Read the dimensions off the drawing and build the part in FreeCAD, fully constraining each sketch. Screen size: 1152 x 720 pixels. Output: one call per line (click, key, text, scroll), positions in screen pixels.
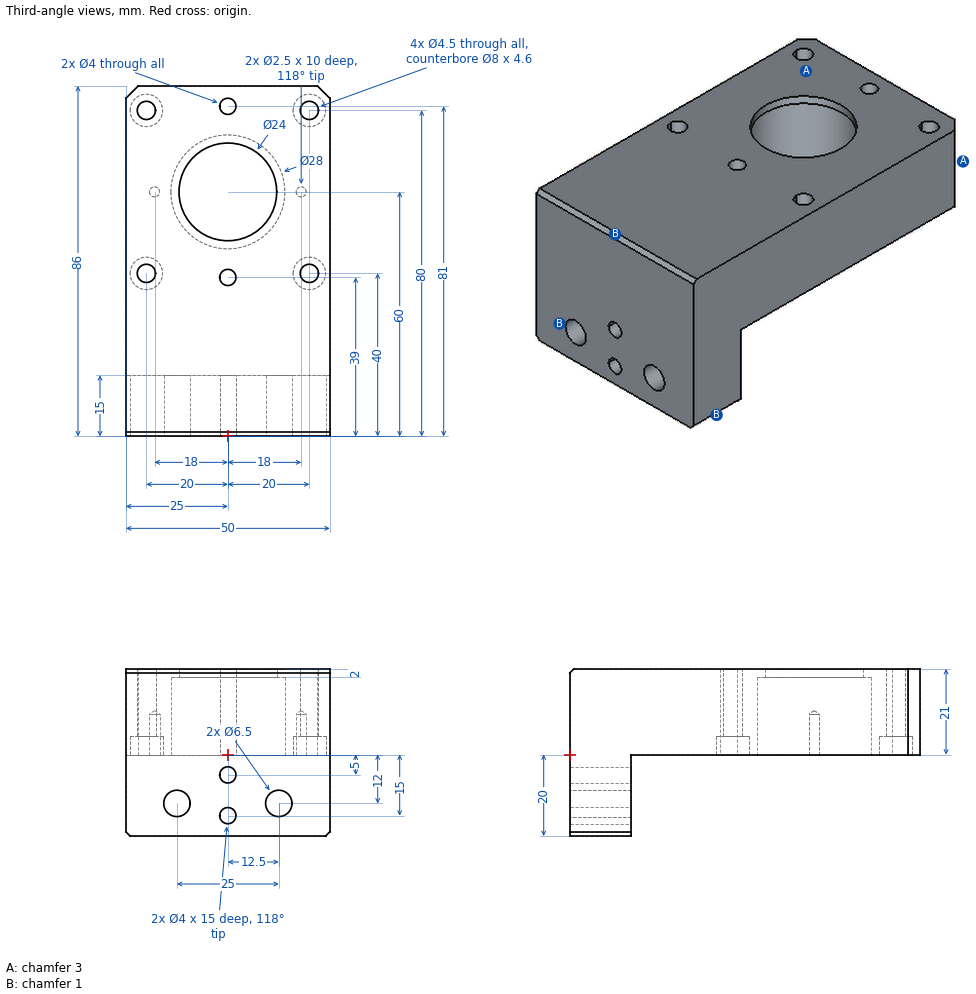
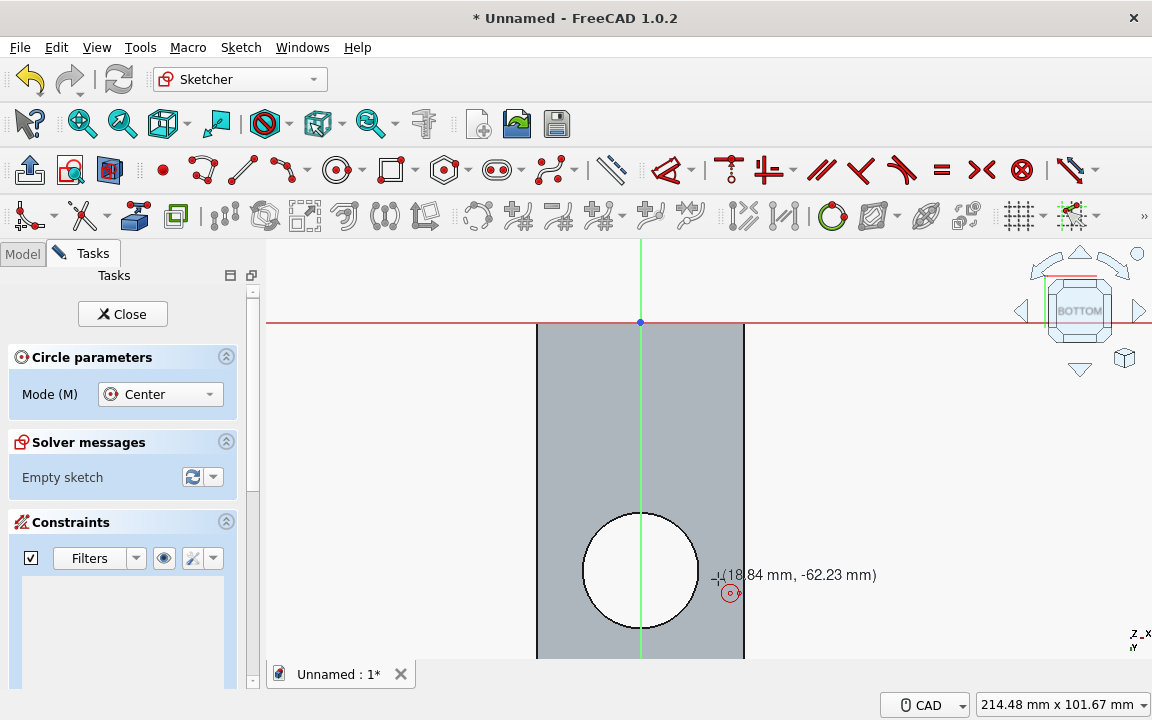
click(715, 571)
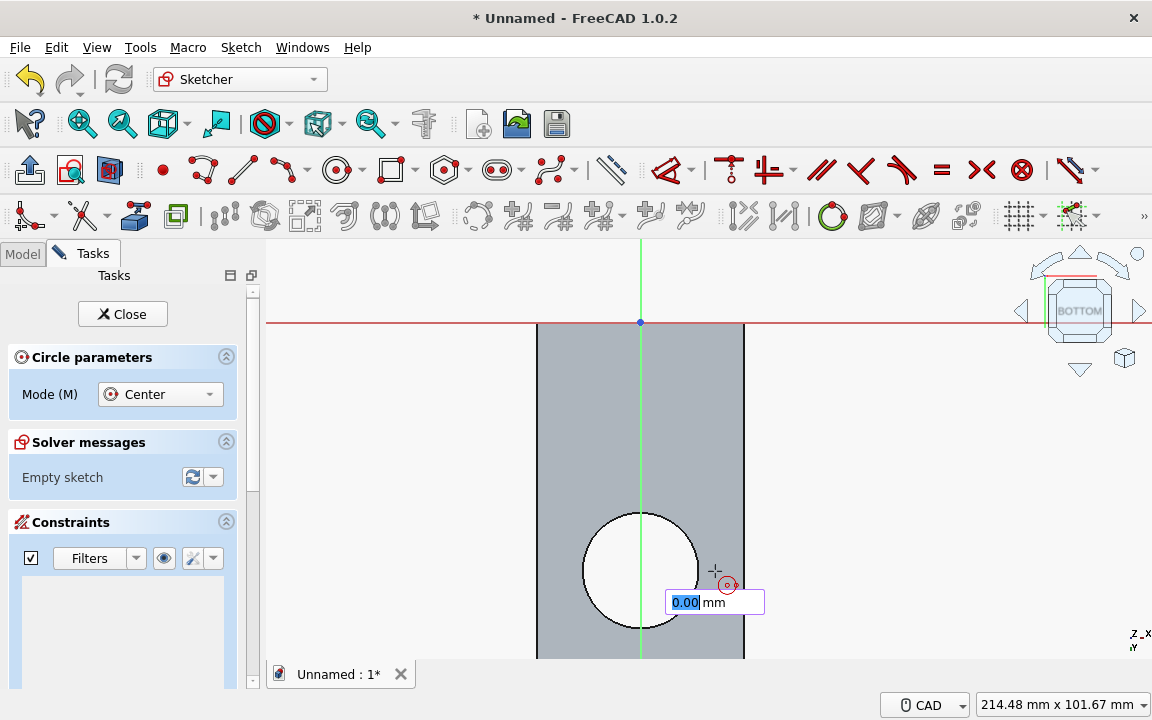
scroll(719, 567, up, 6)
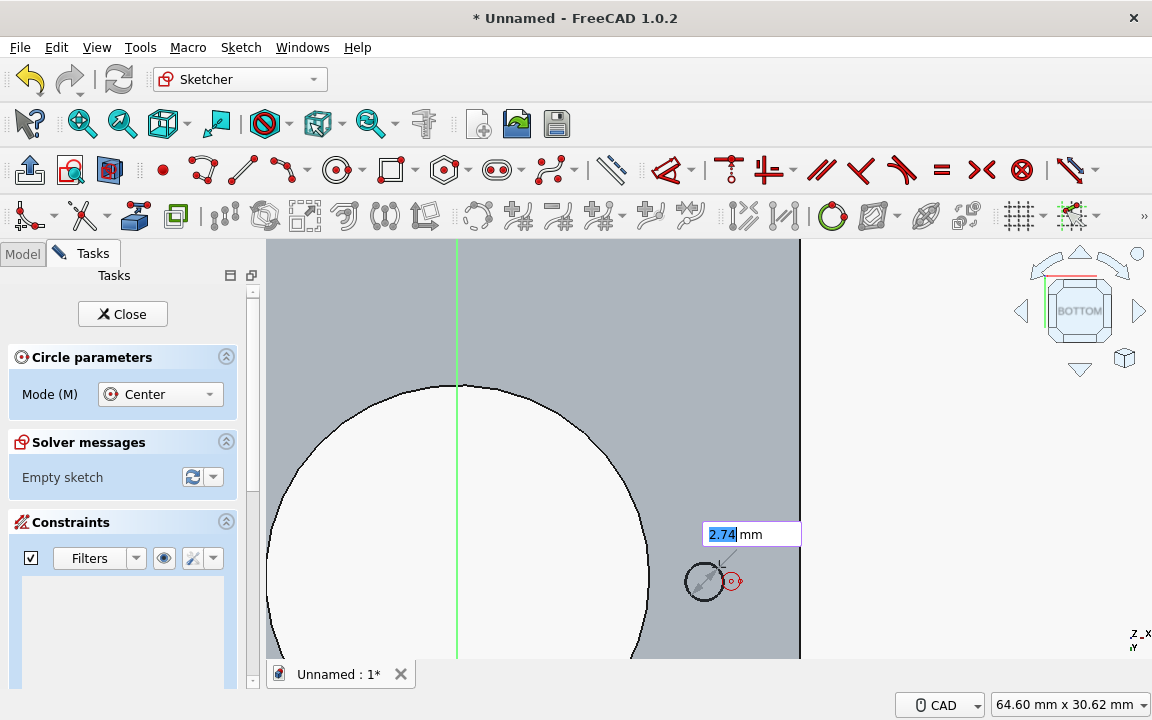
click(716, 565)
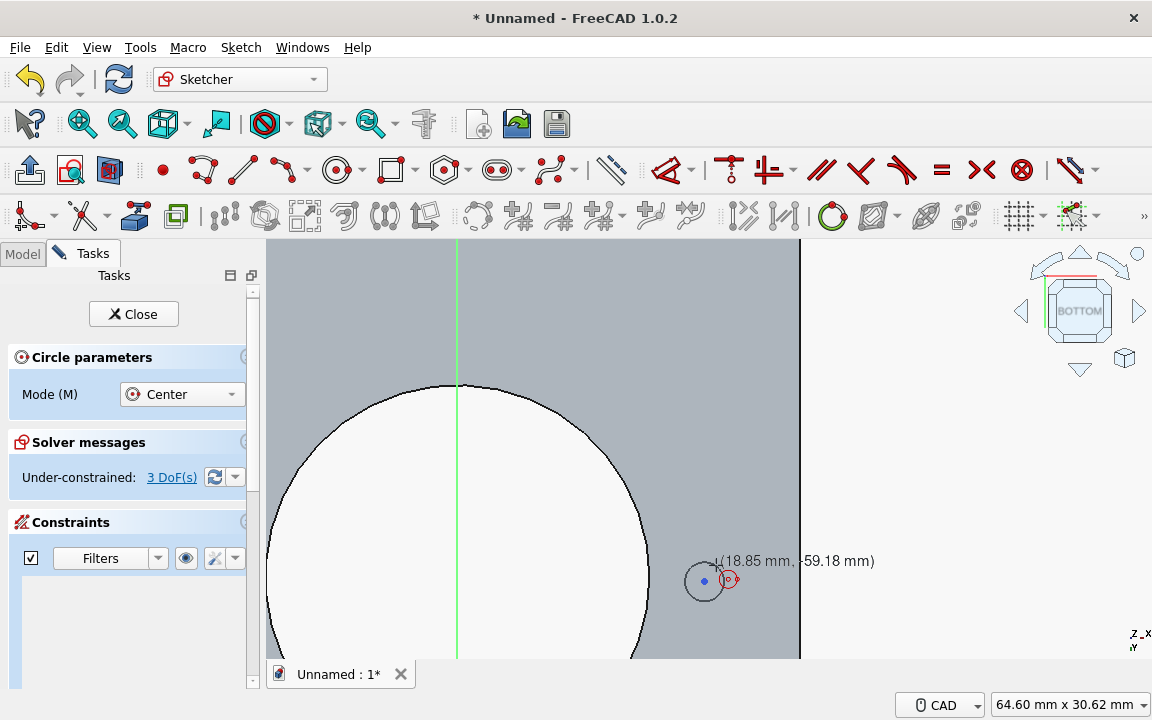
scroll(719, 567, down, 6)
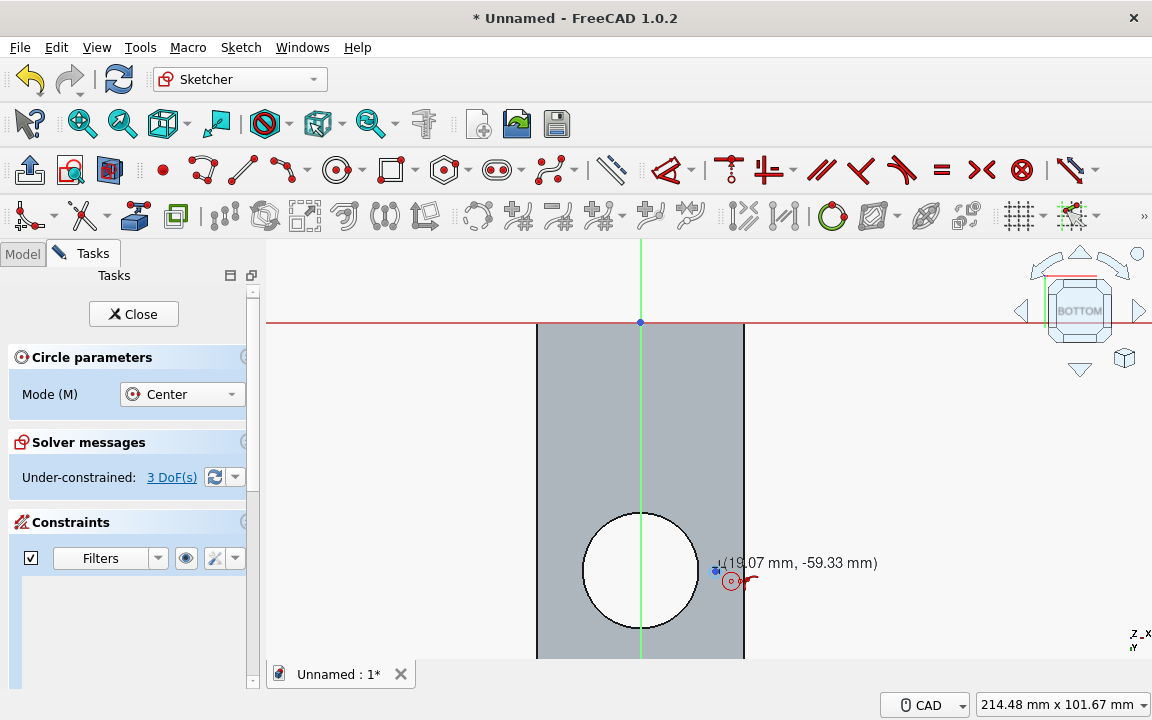
scroll(566, 571, up, 8)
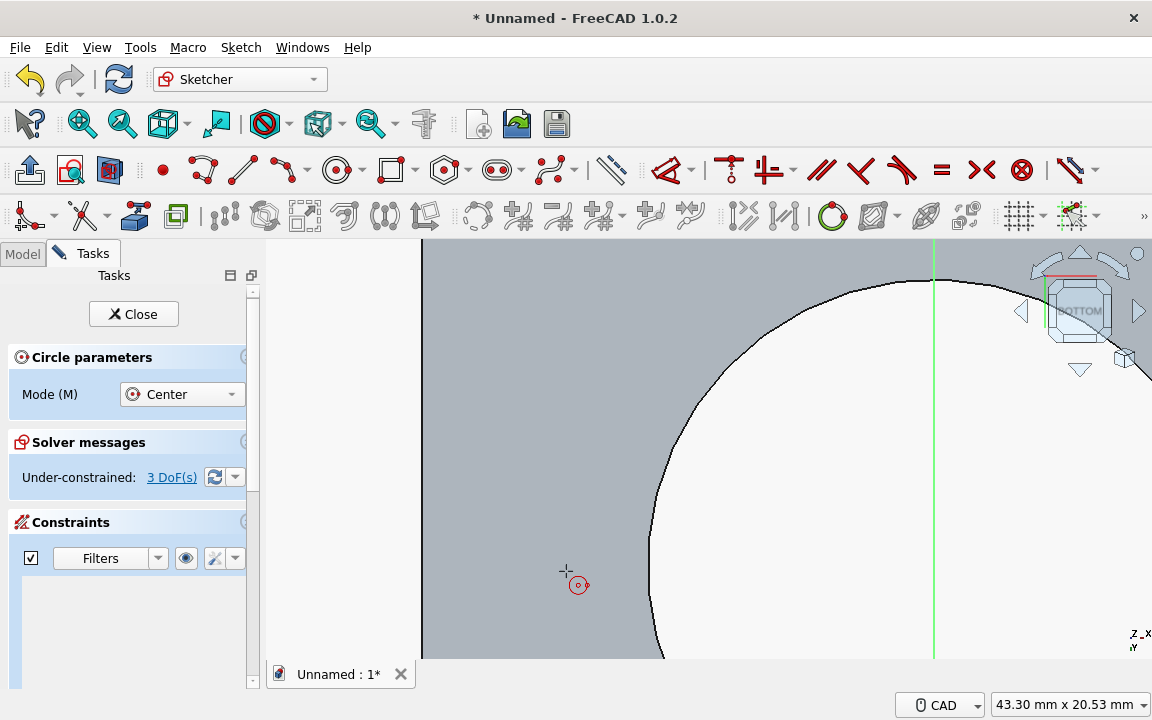
scroll(566, 571, down, 8)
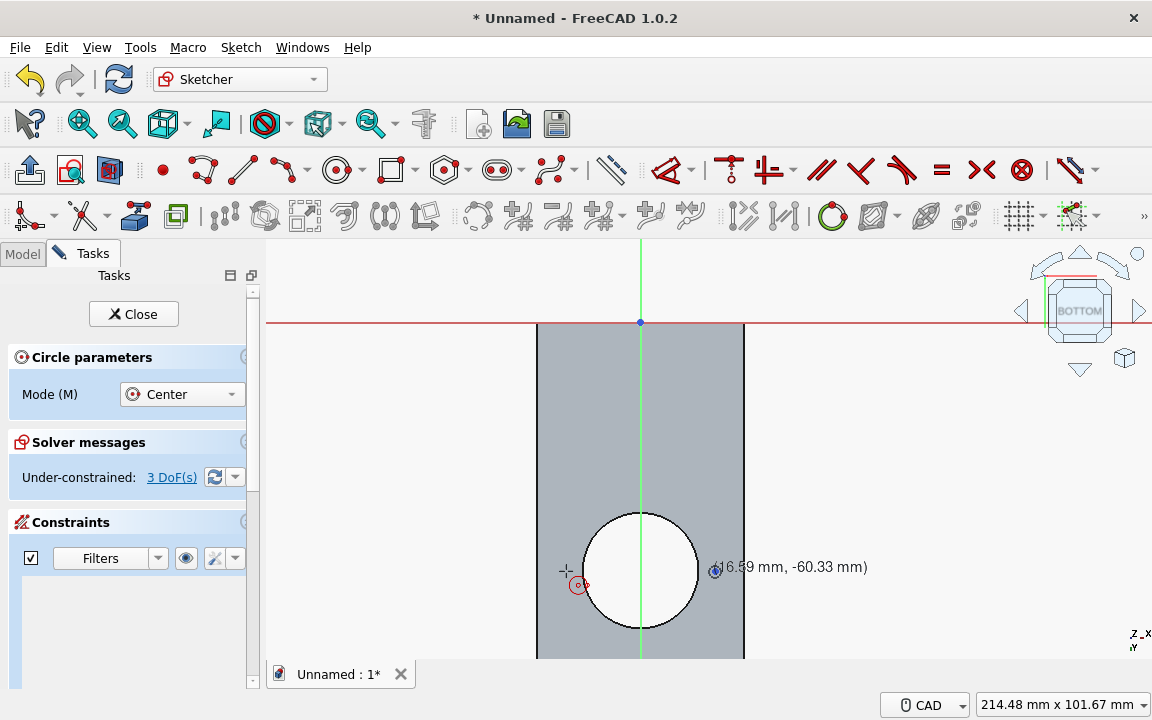
click(566, 571)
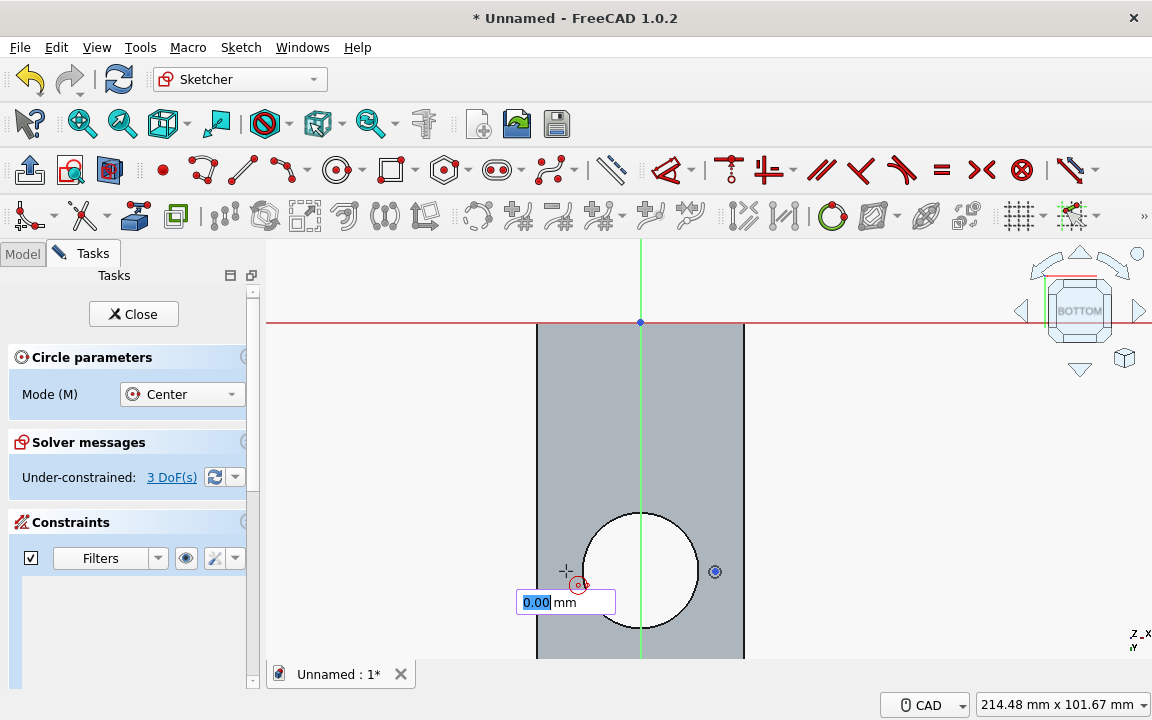
scroll(570, 567, up, 6)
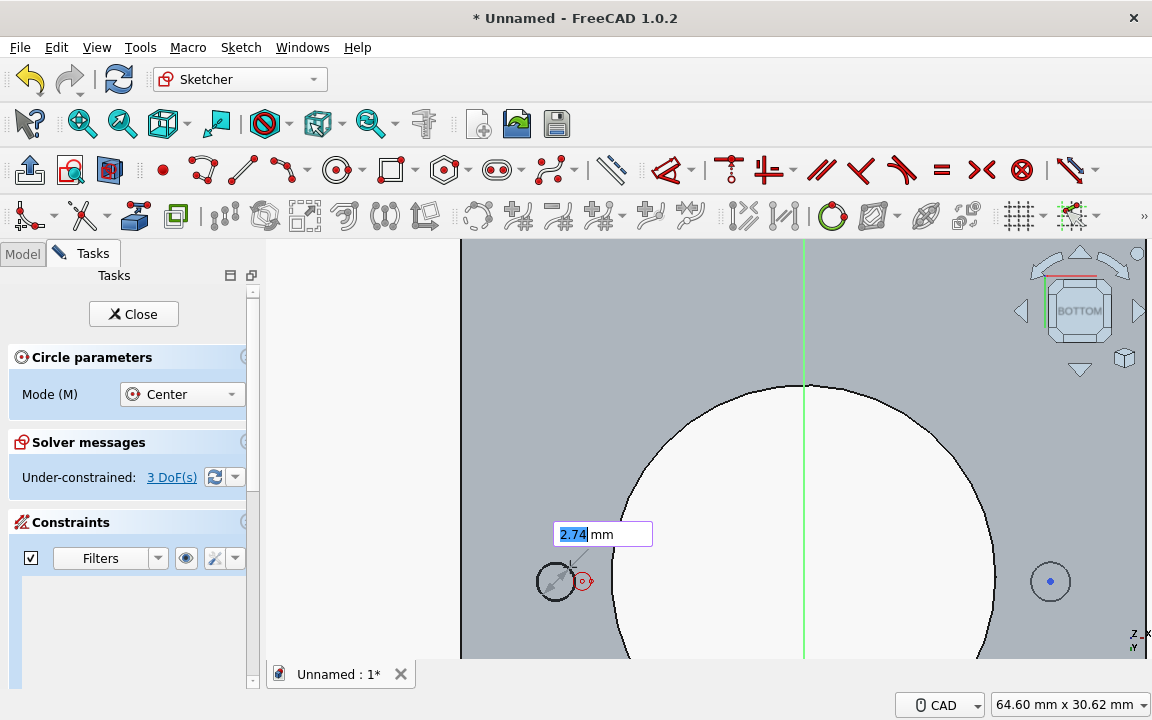
click(569, 565)
key(Escape)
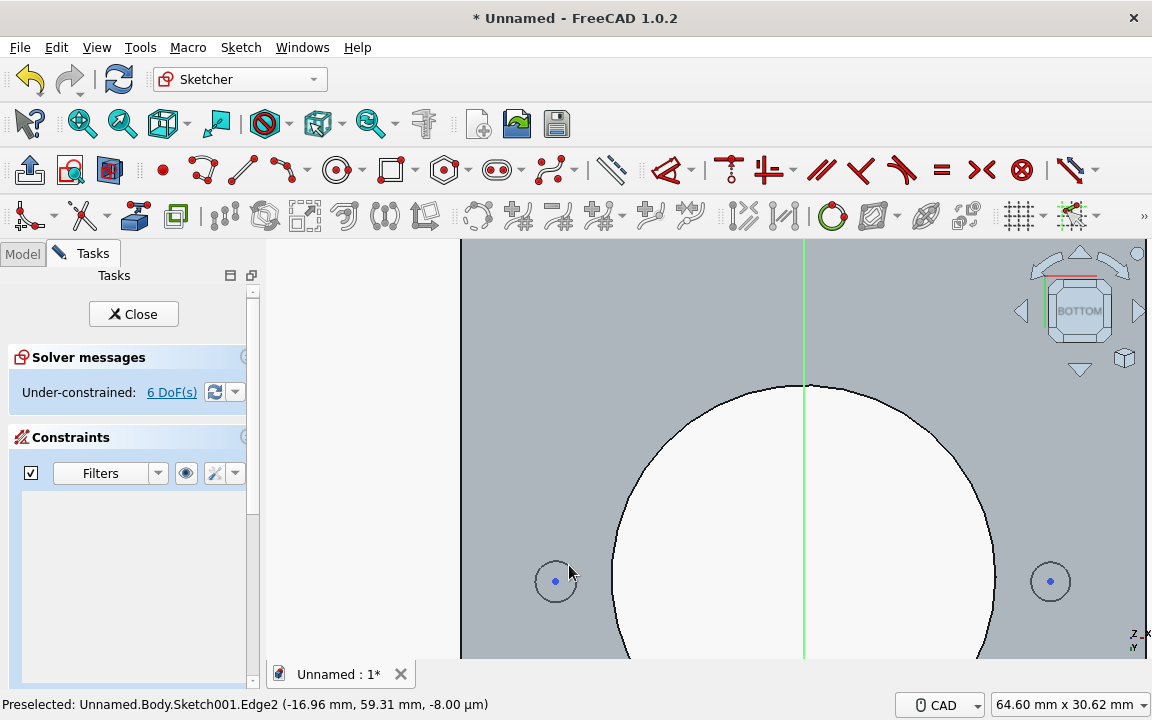
scroll(570, 567, down, 6)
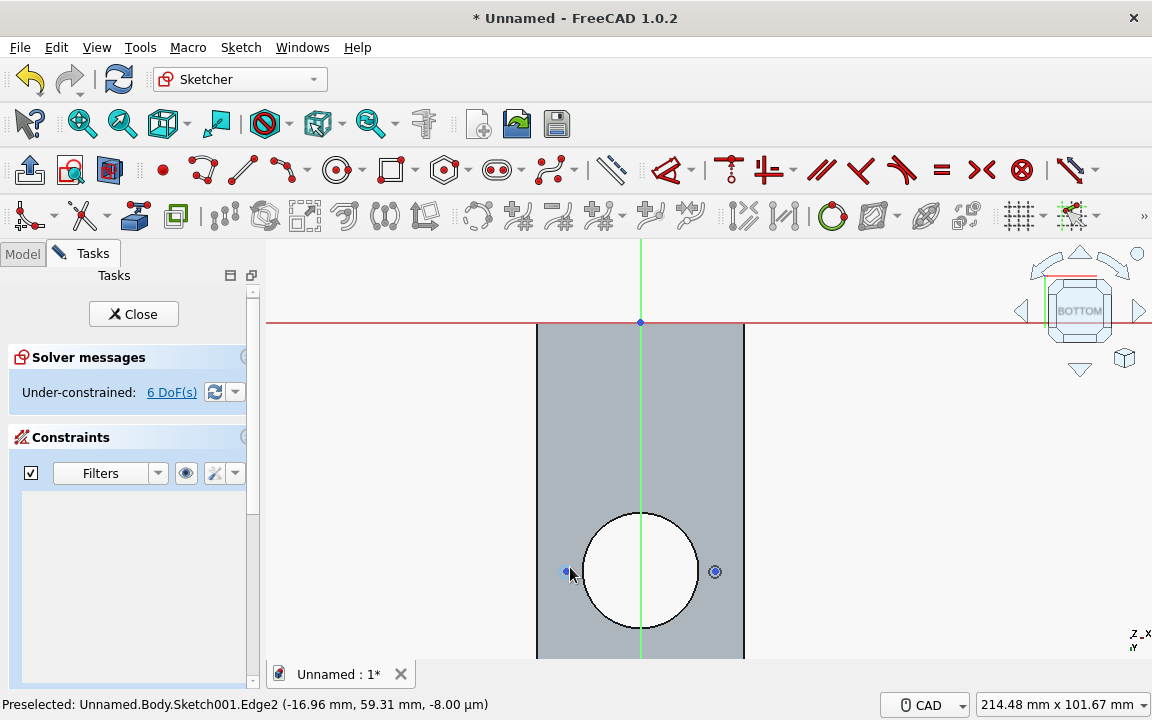
scroll(719, 568, up, 5)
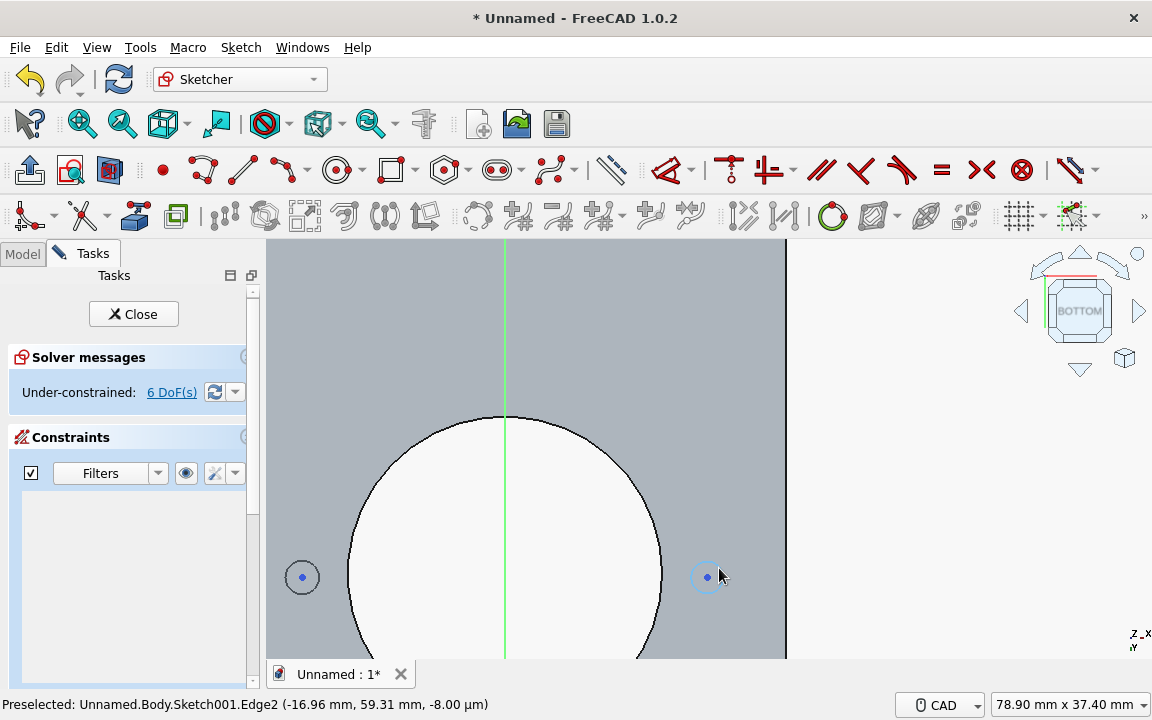
click(719, 566)